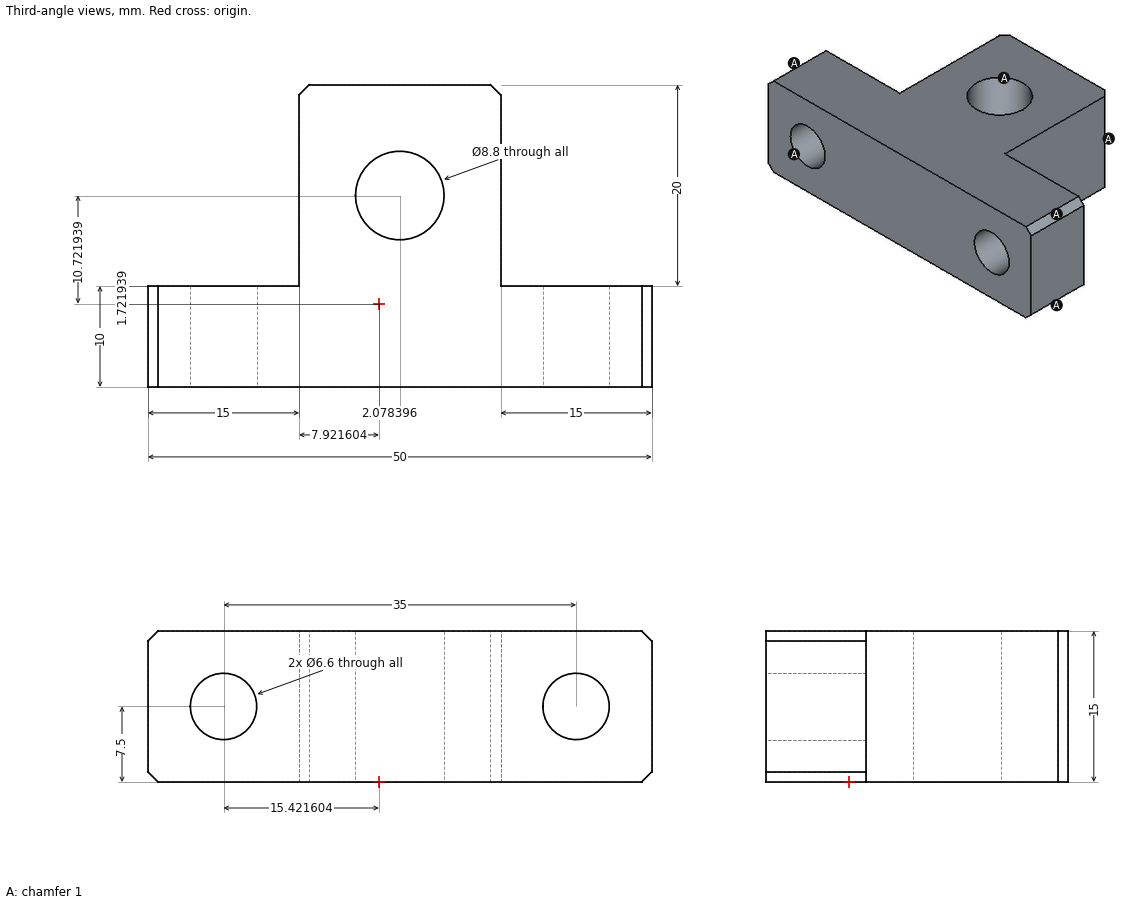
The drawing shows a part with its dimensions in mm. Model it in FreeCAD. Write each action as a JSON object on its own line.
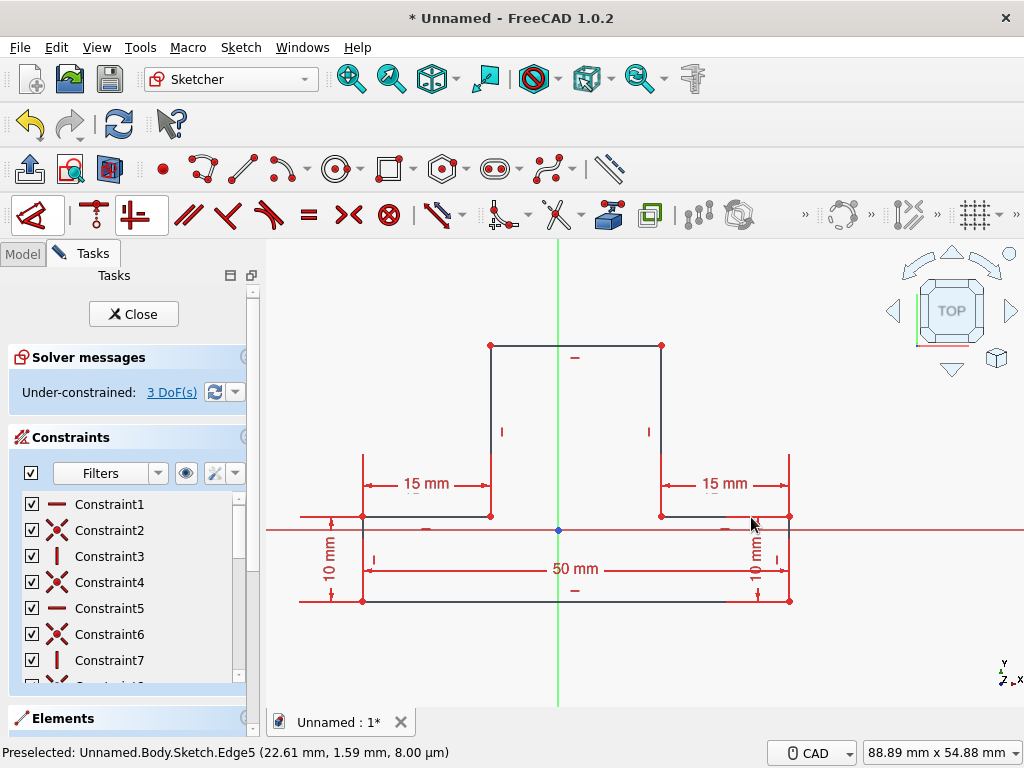
{"action": "left_click", "coordinate": [661, 466]}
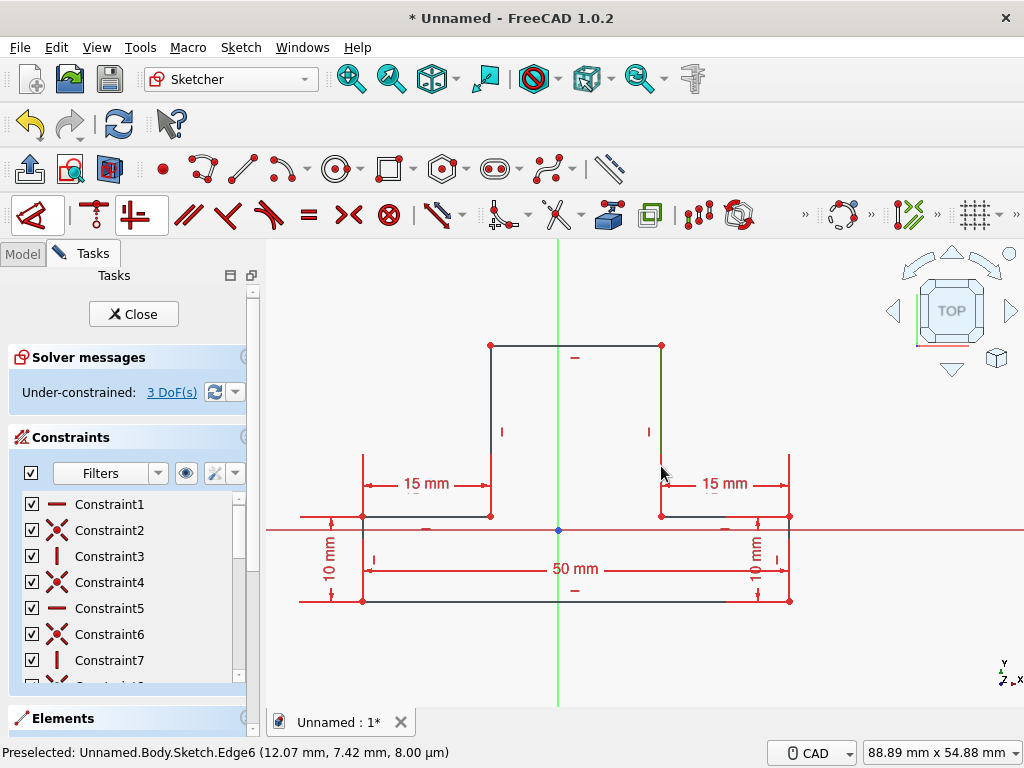
{"action": "key", "text": "i"}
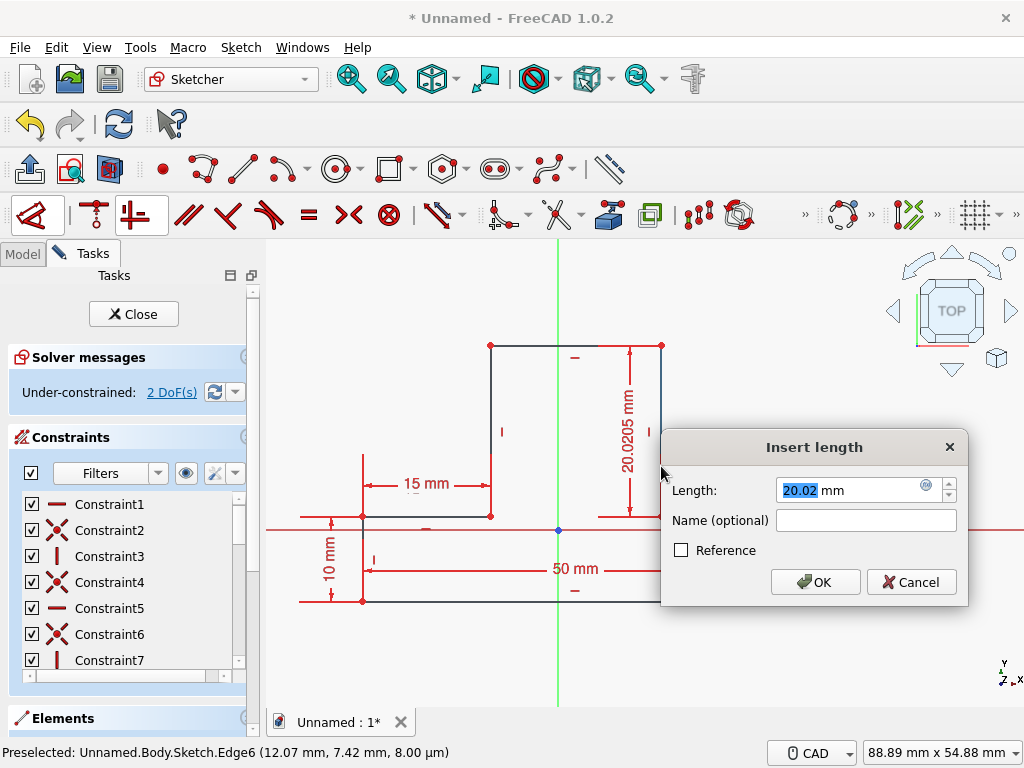
{"action": "type", "text": "20"}
{"action": "key", "text": "Return"}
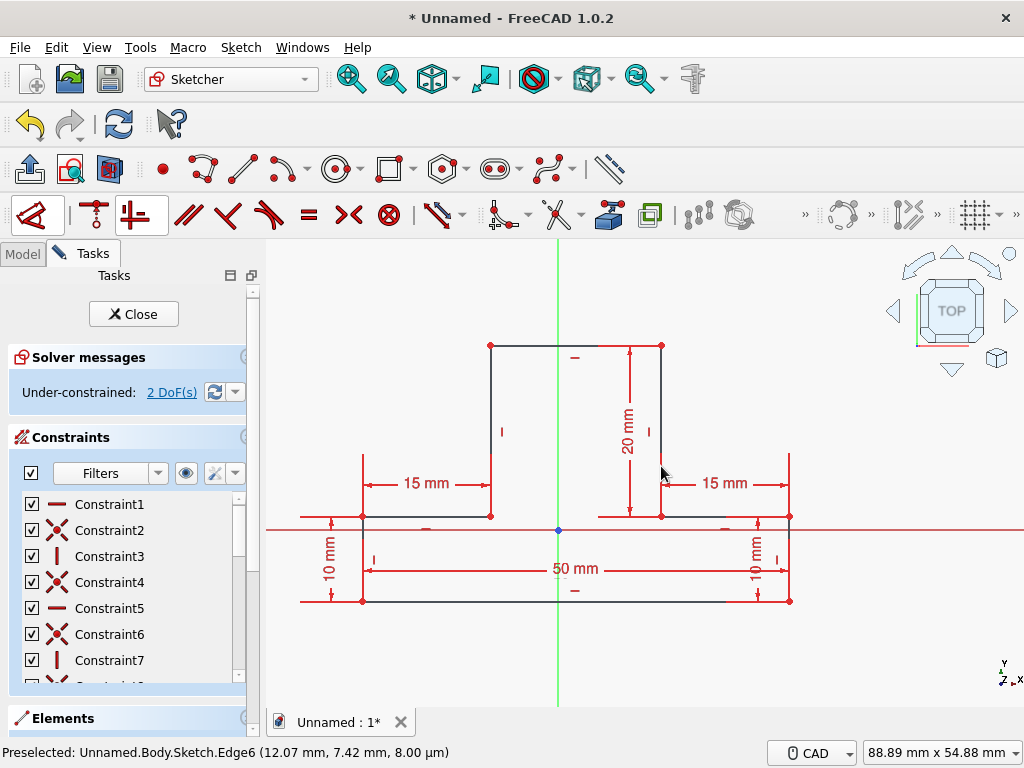
{"action": "left_click", "coordinate": [491, 517]}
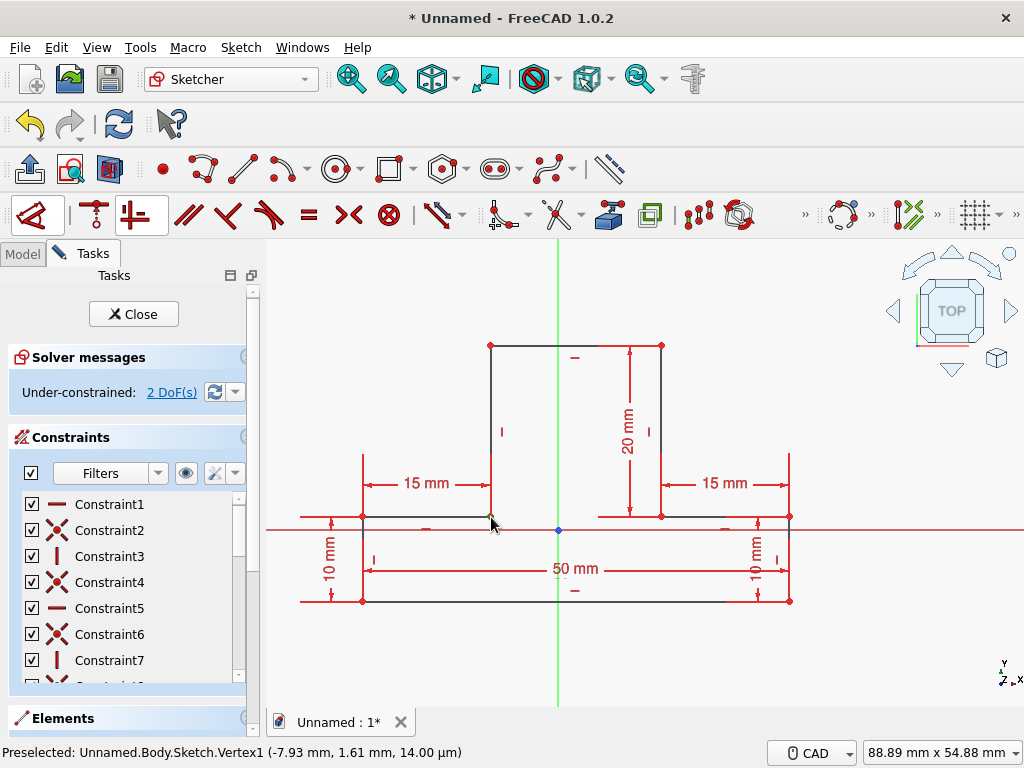
{"action": "left_click", "coordinate": [58, 216]}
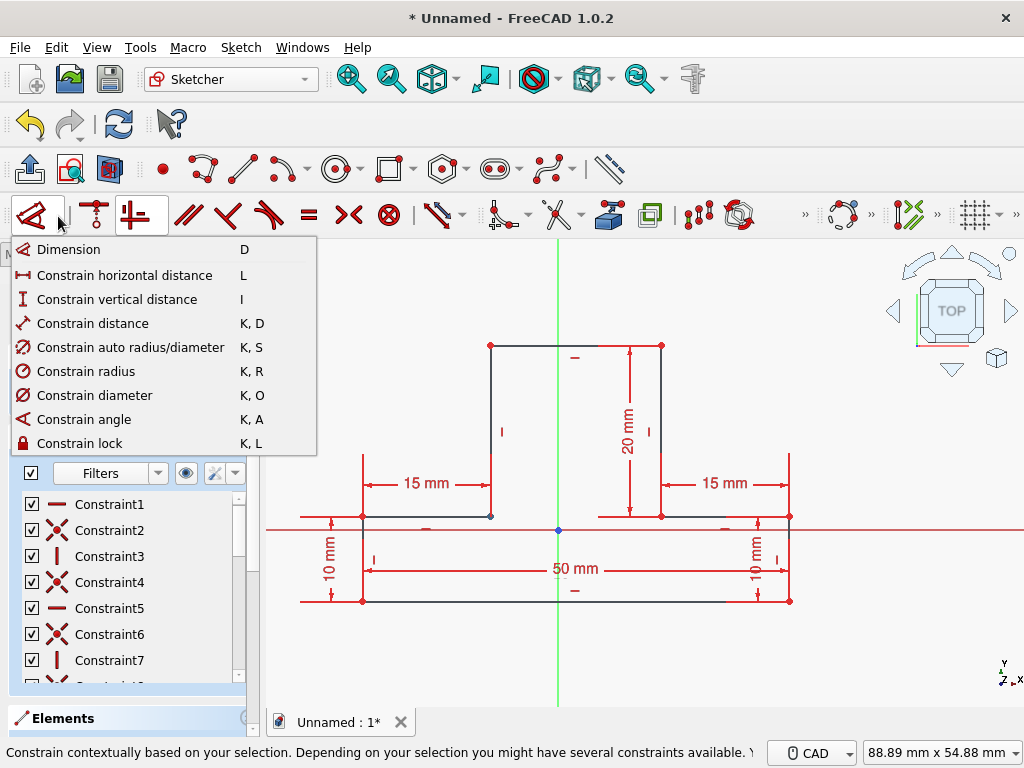
{"action": "left_click", "coordinate": [164, 275]}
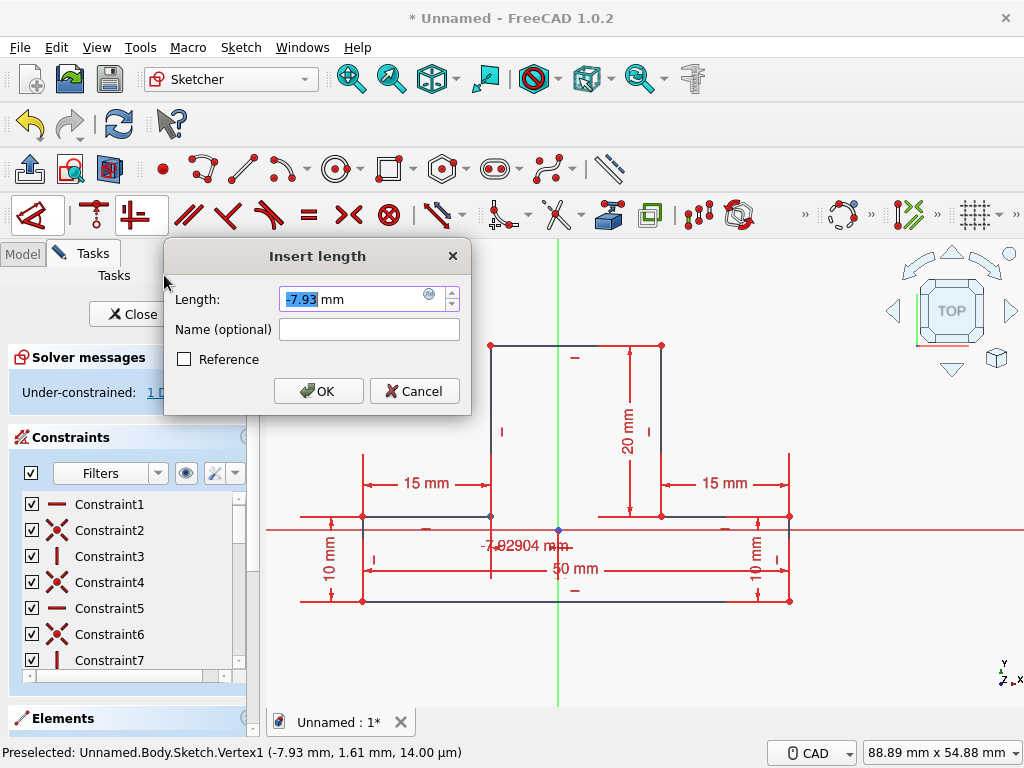
{"action": "type", "text": "-7.921604"}
{"action": "key", "text": "Return"}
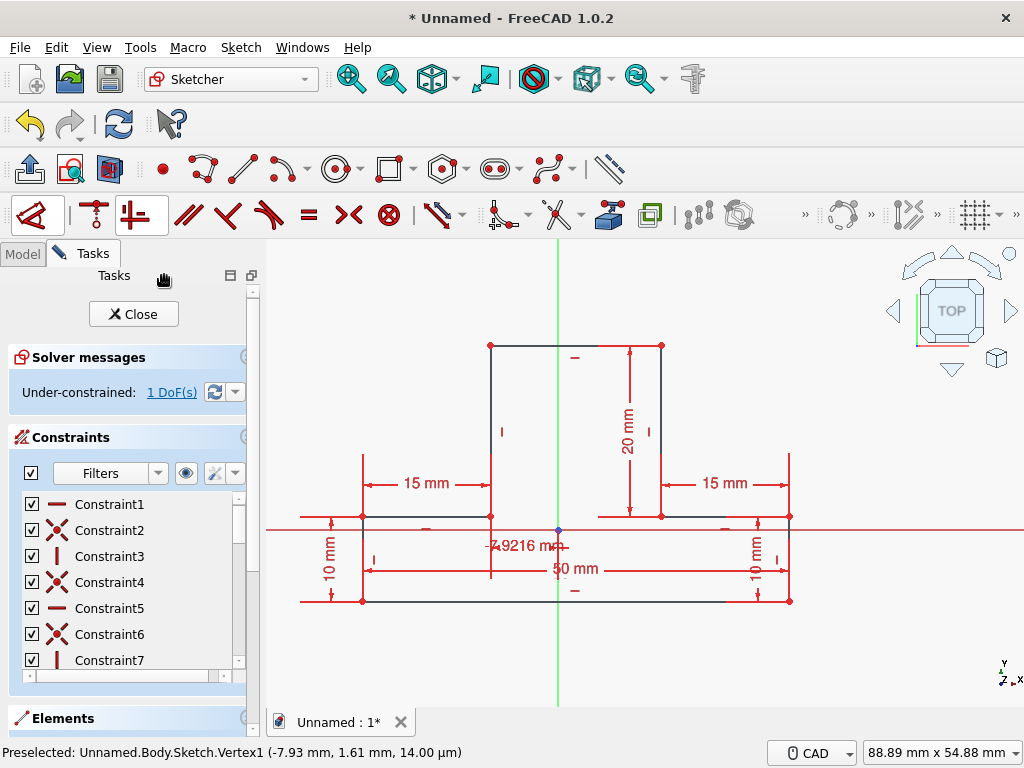
{"action": "scroll", "coordinate": [491, 517], "scroll_direction": "up", "scroll_amount": 5}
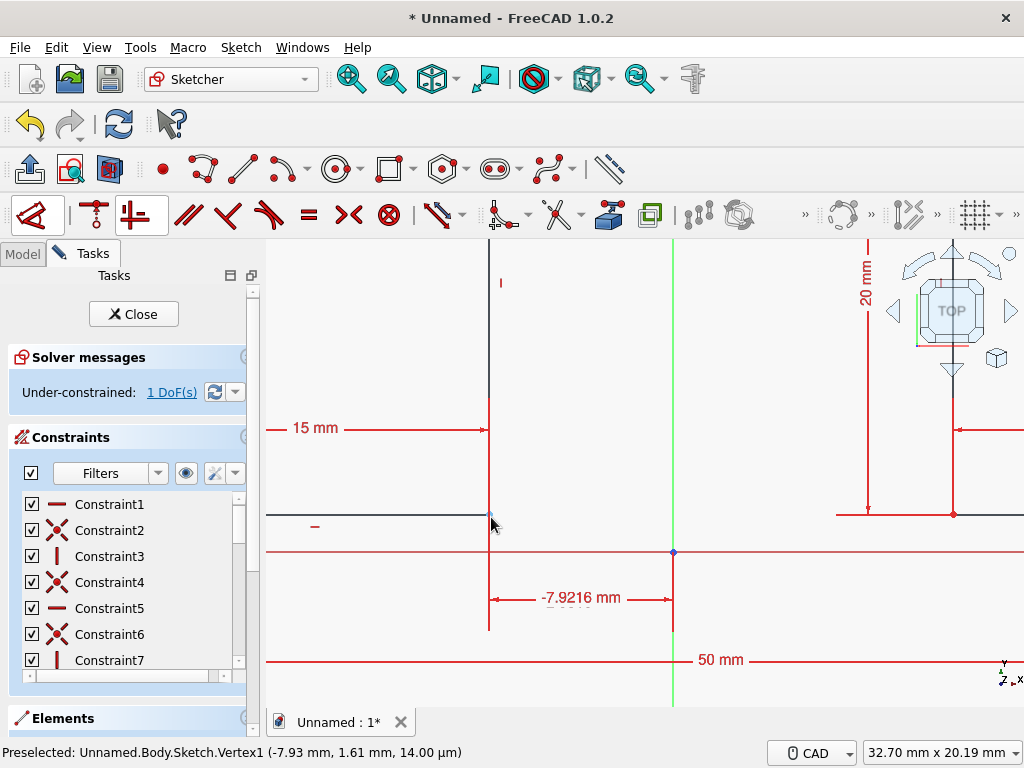
{"action": "left_click", "coordinate": [489, 515]}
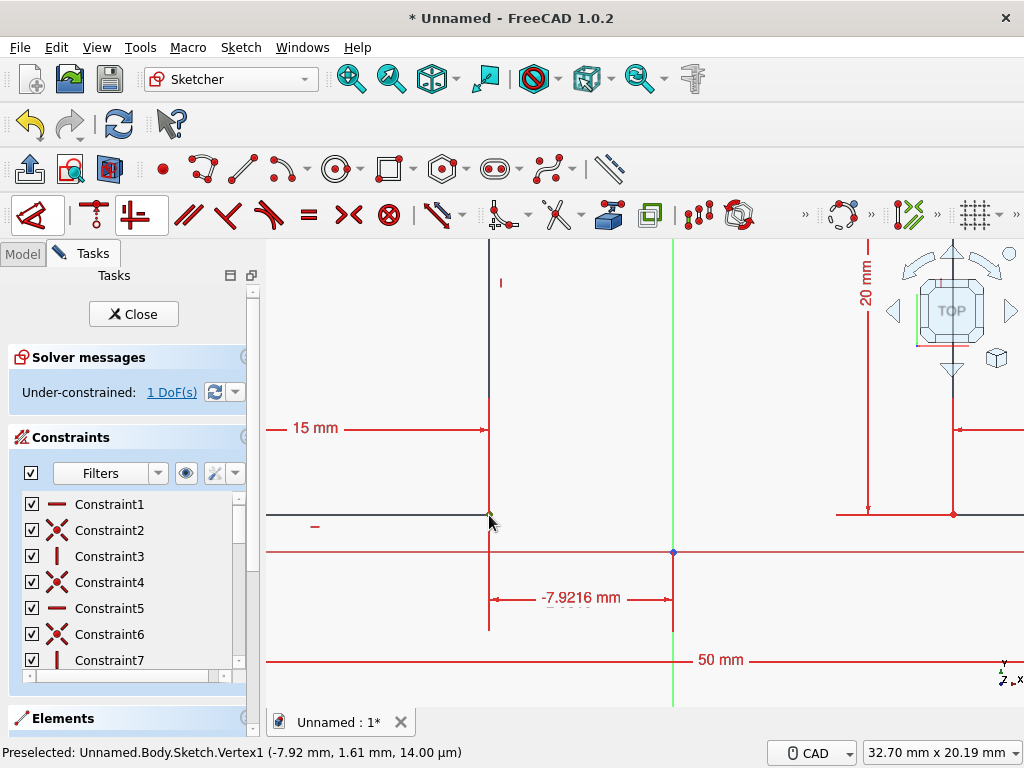
{"action": "left_click", "coordinate": [58, 216]}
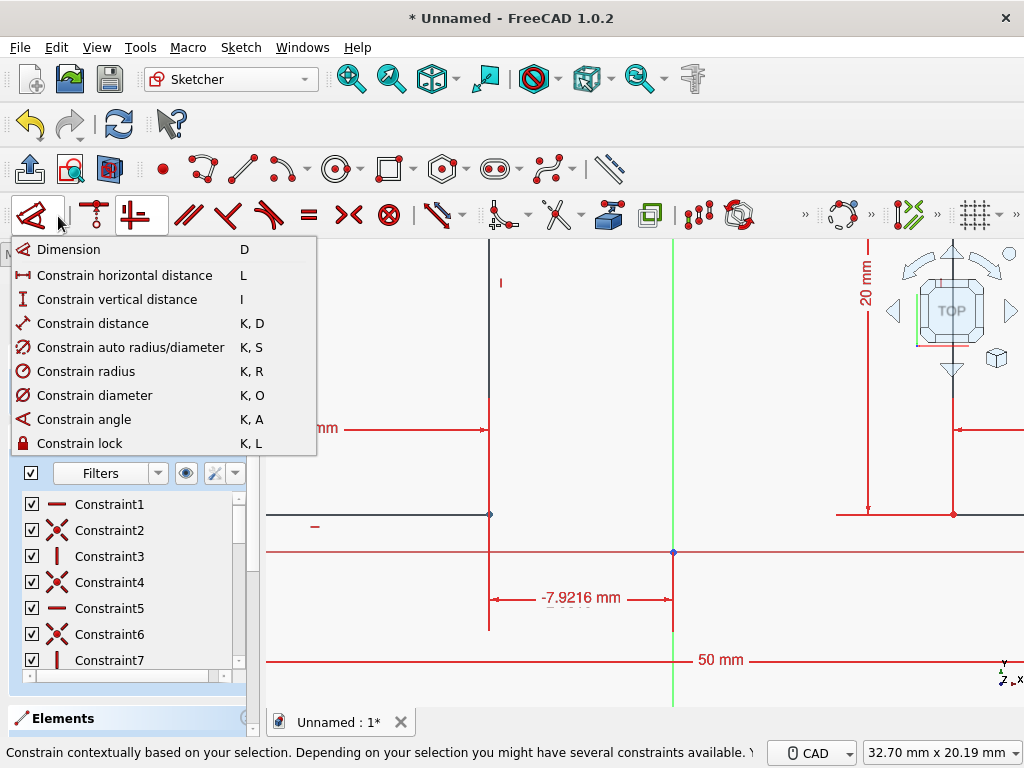
{"action": "left_click", "coordinate": [164, 299]}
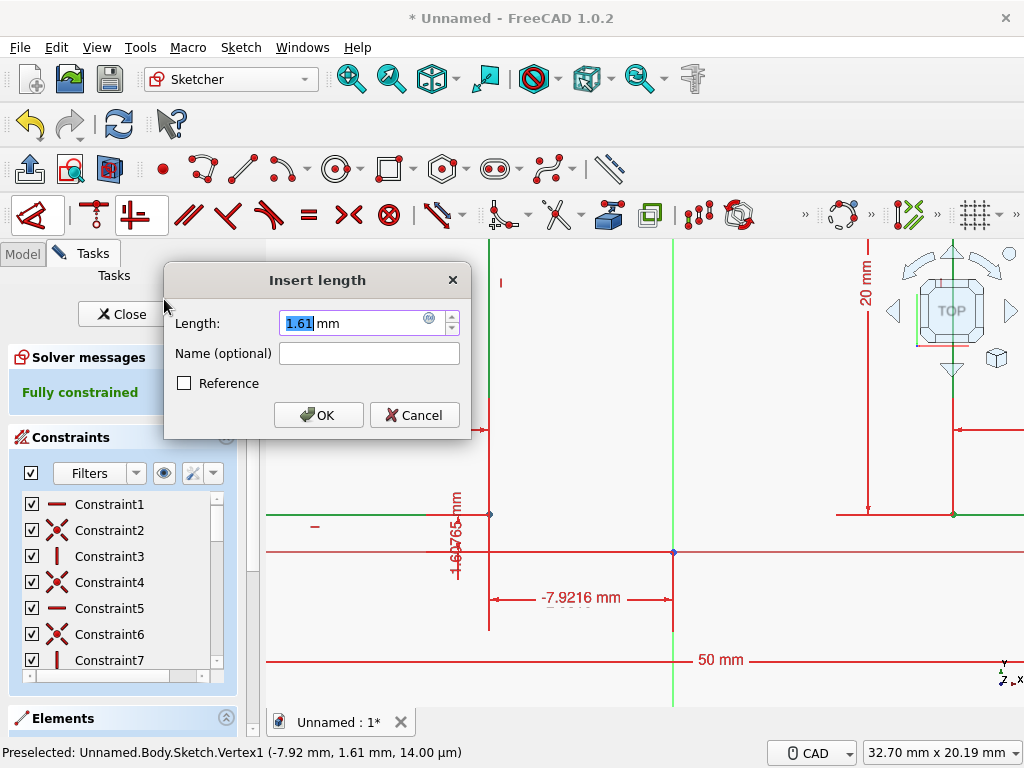
{"action": "type", "text": "1.721939"}
{"action": "key", "text": "Return"}